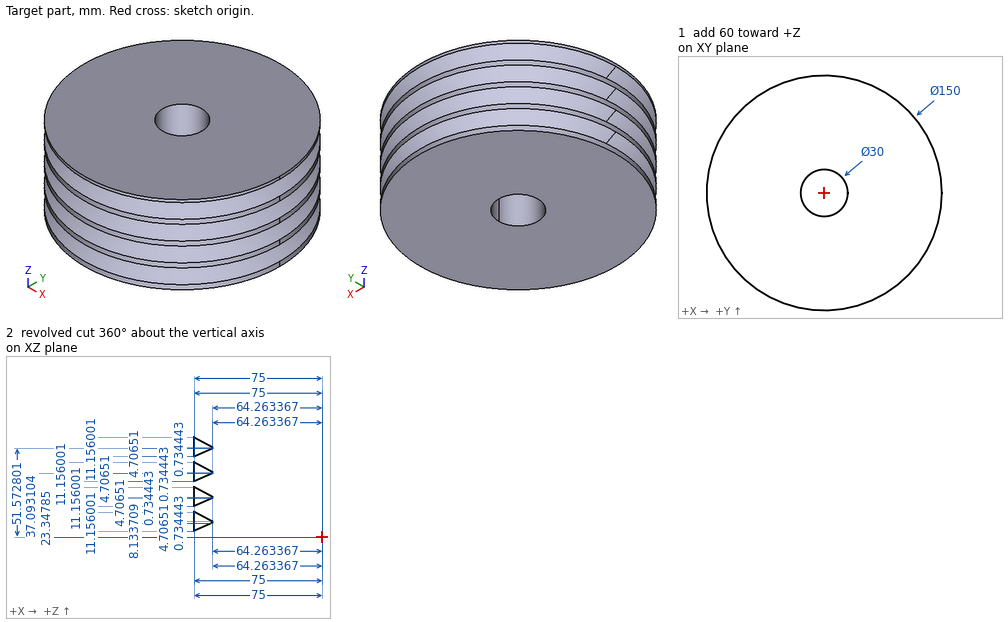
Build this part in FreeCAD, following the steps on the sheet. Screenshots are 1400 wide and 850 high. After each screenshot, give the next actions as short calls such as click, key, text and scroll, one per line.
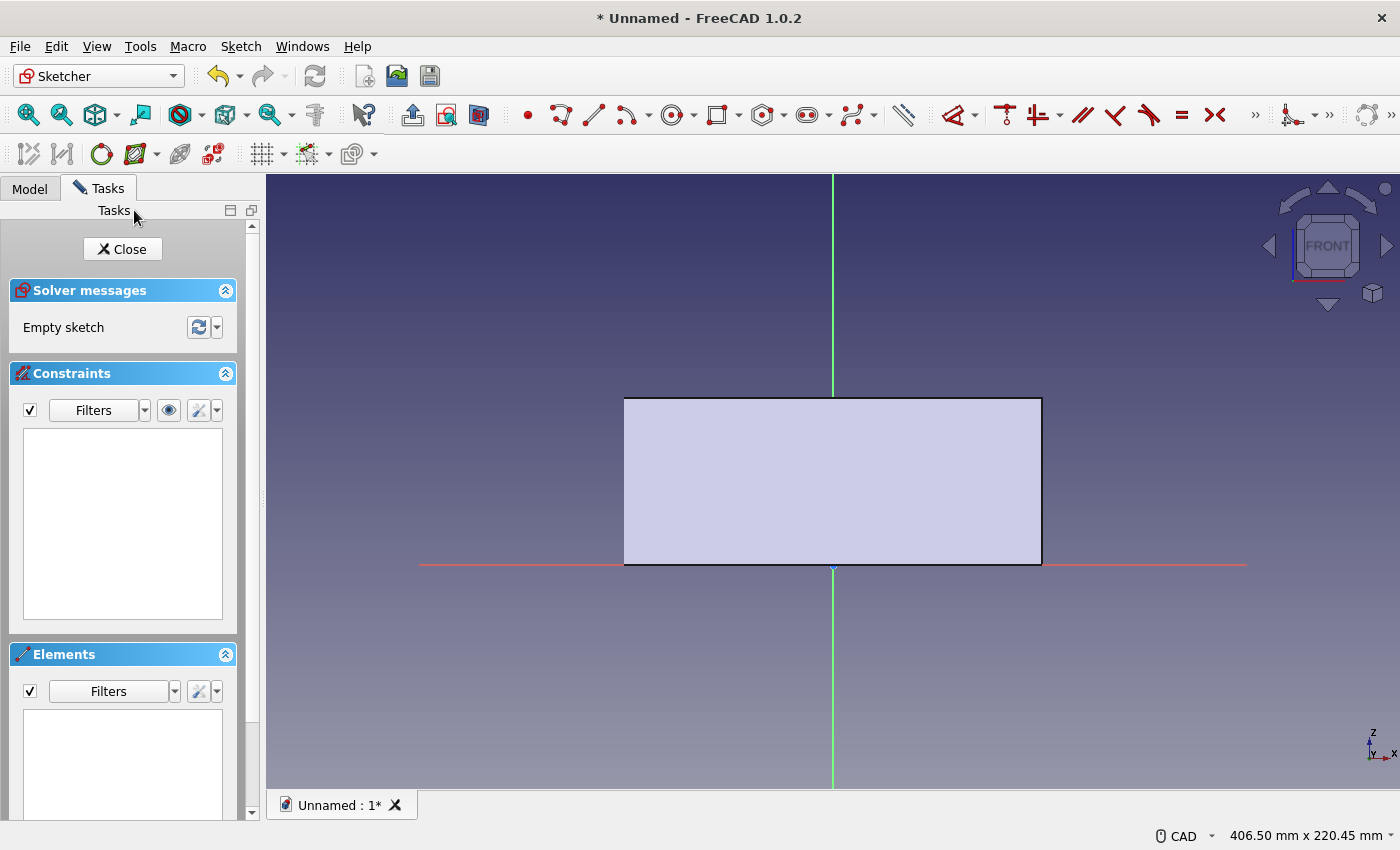
click(479, 116)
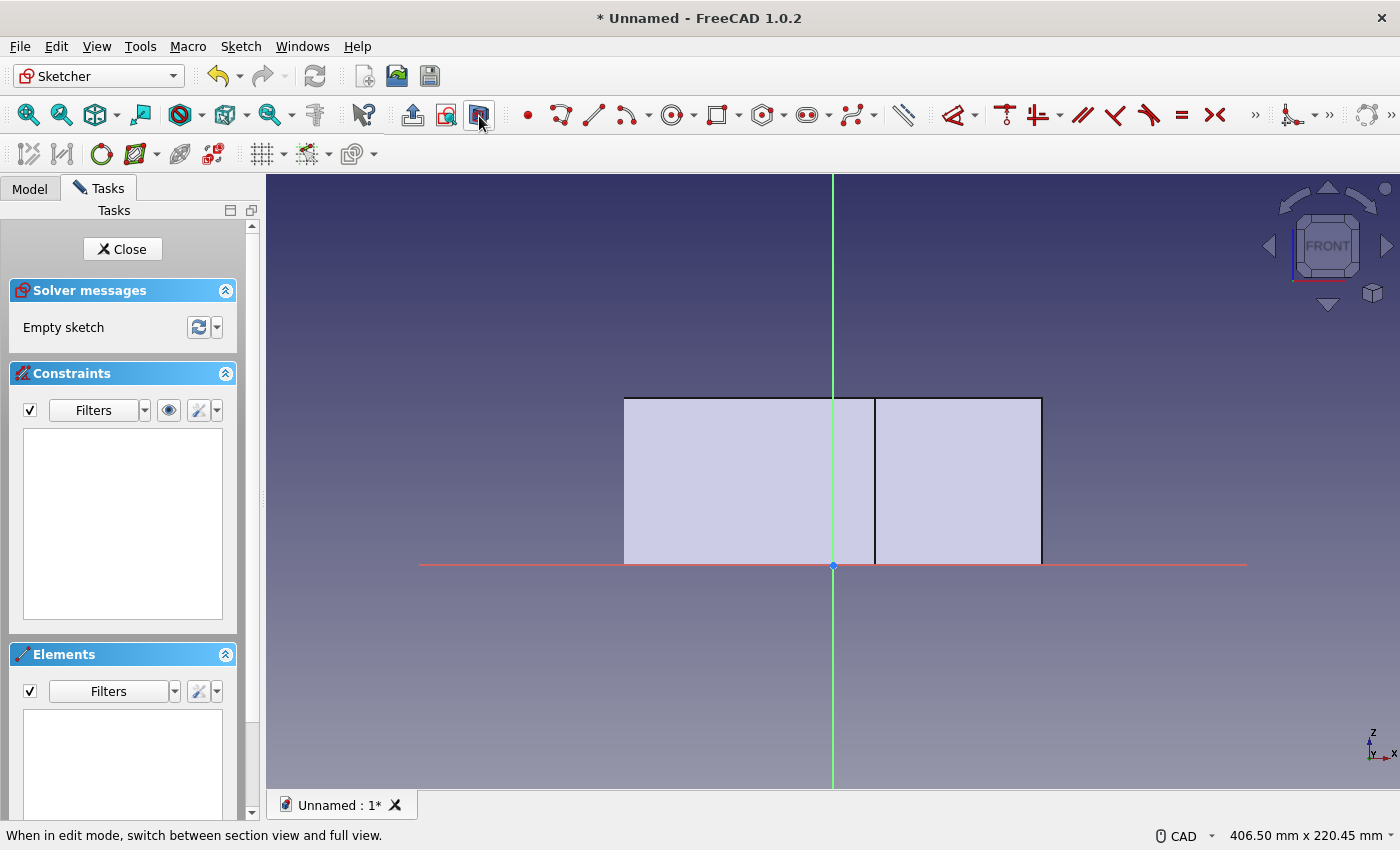
scroll(699, 487, up, 4)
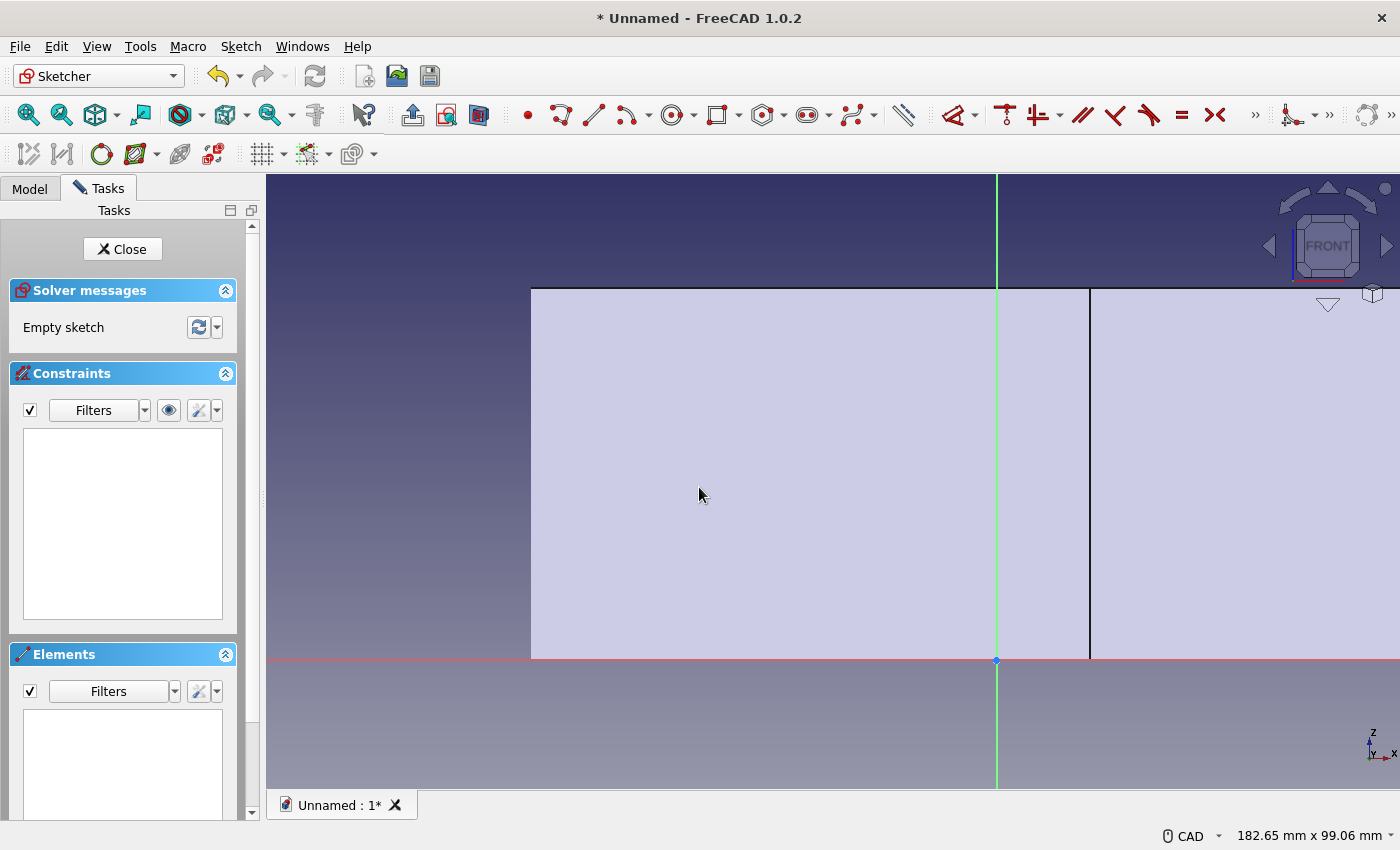
click(561, 116)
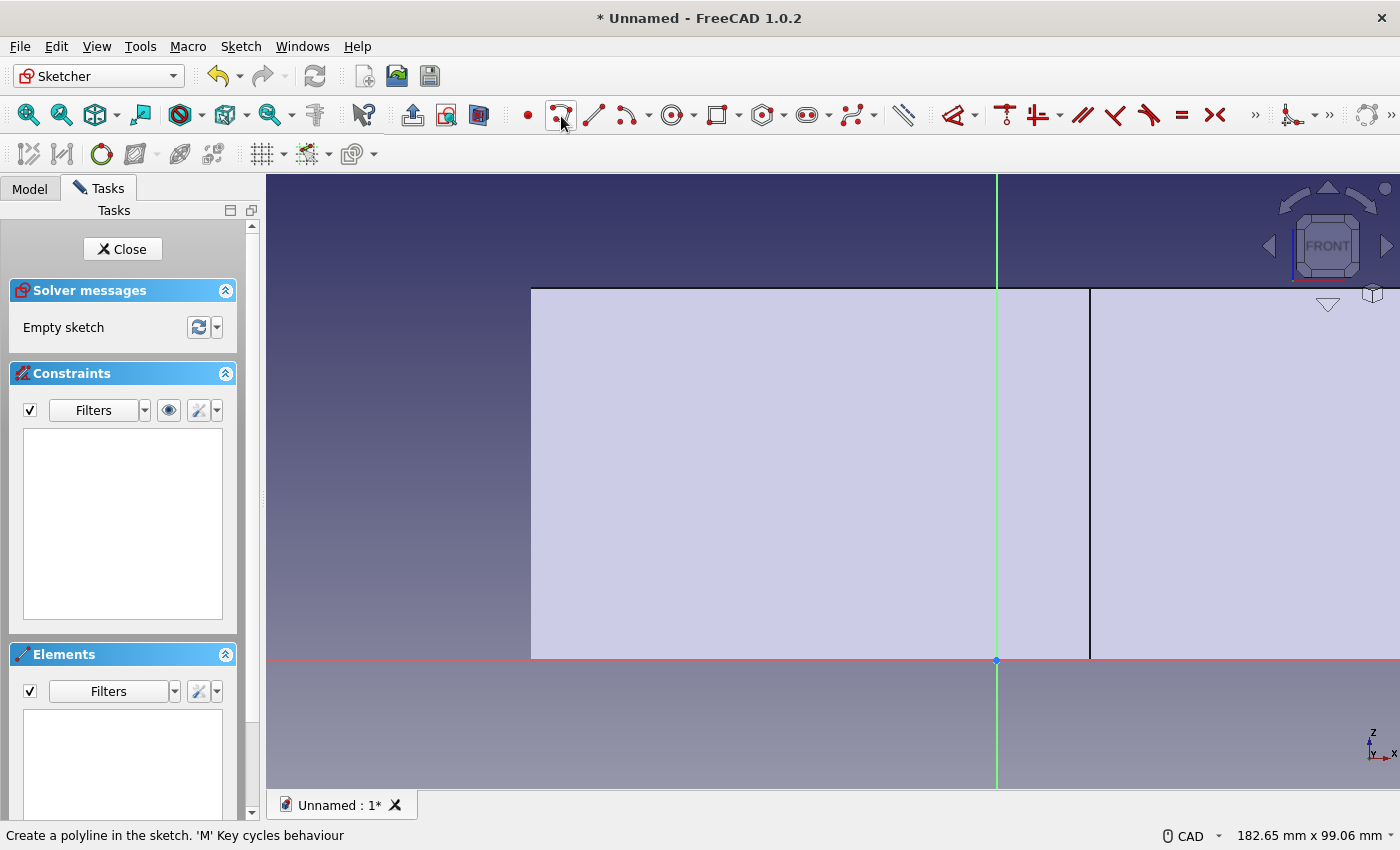
click(598, 340)
click(531, 369)
click(531, 300)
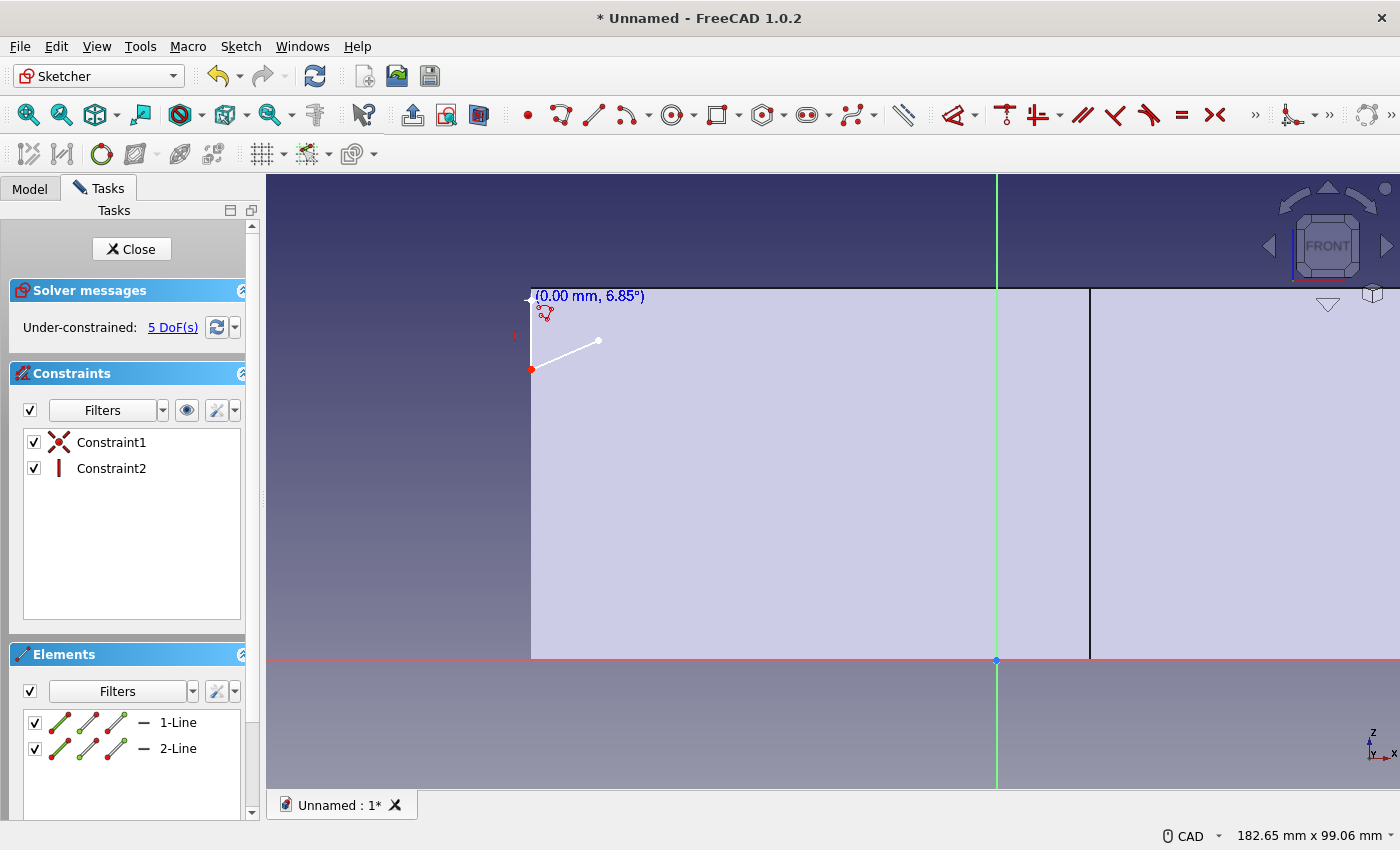
scroll(598, 336, up, 7)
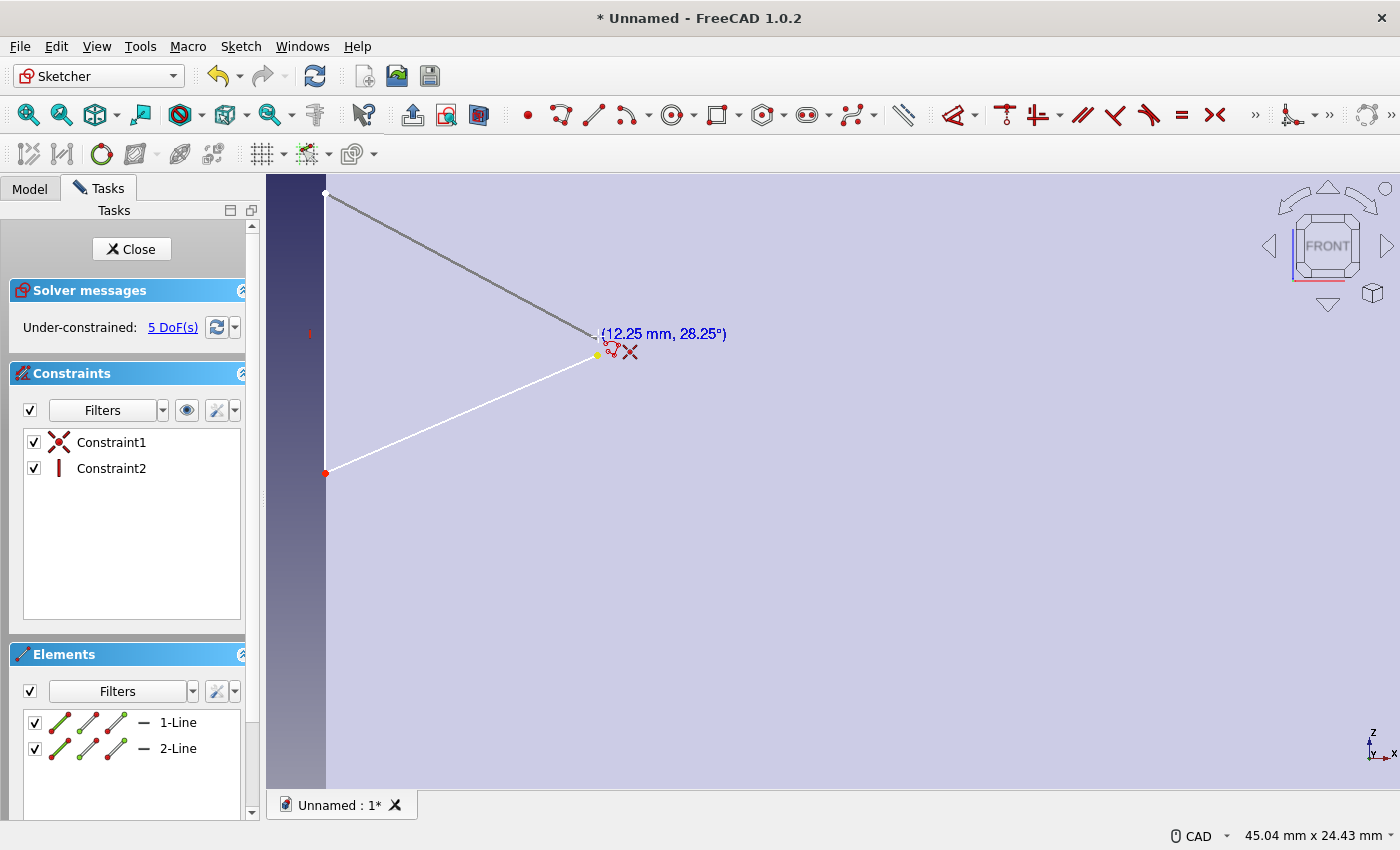
click(596, 334)
click(597, 355)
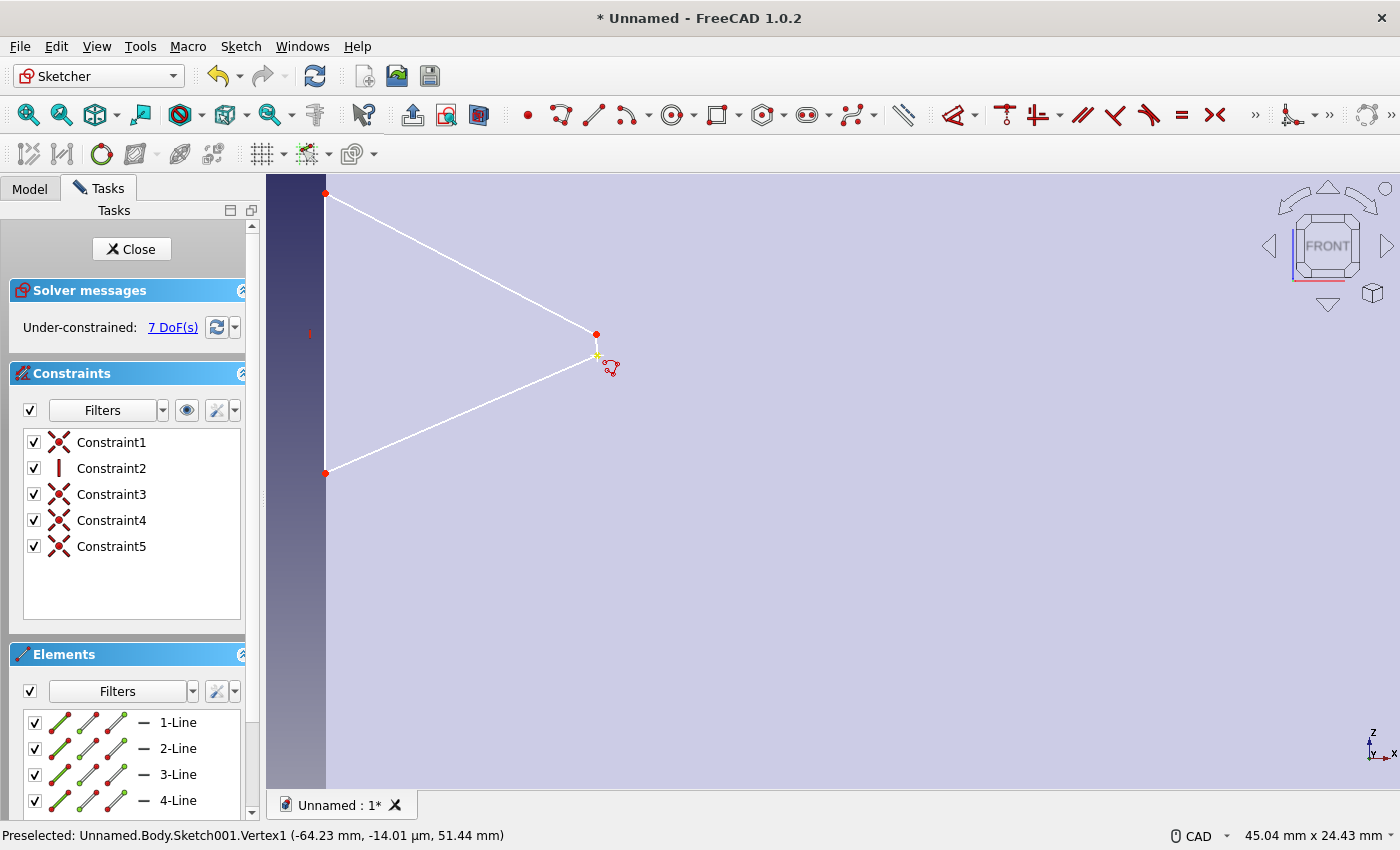
scroll(599, 338, down, 7)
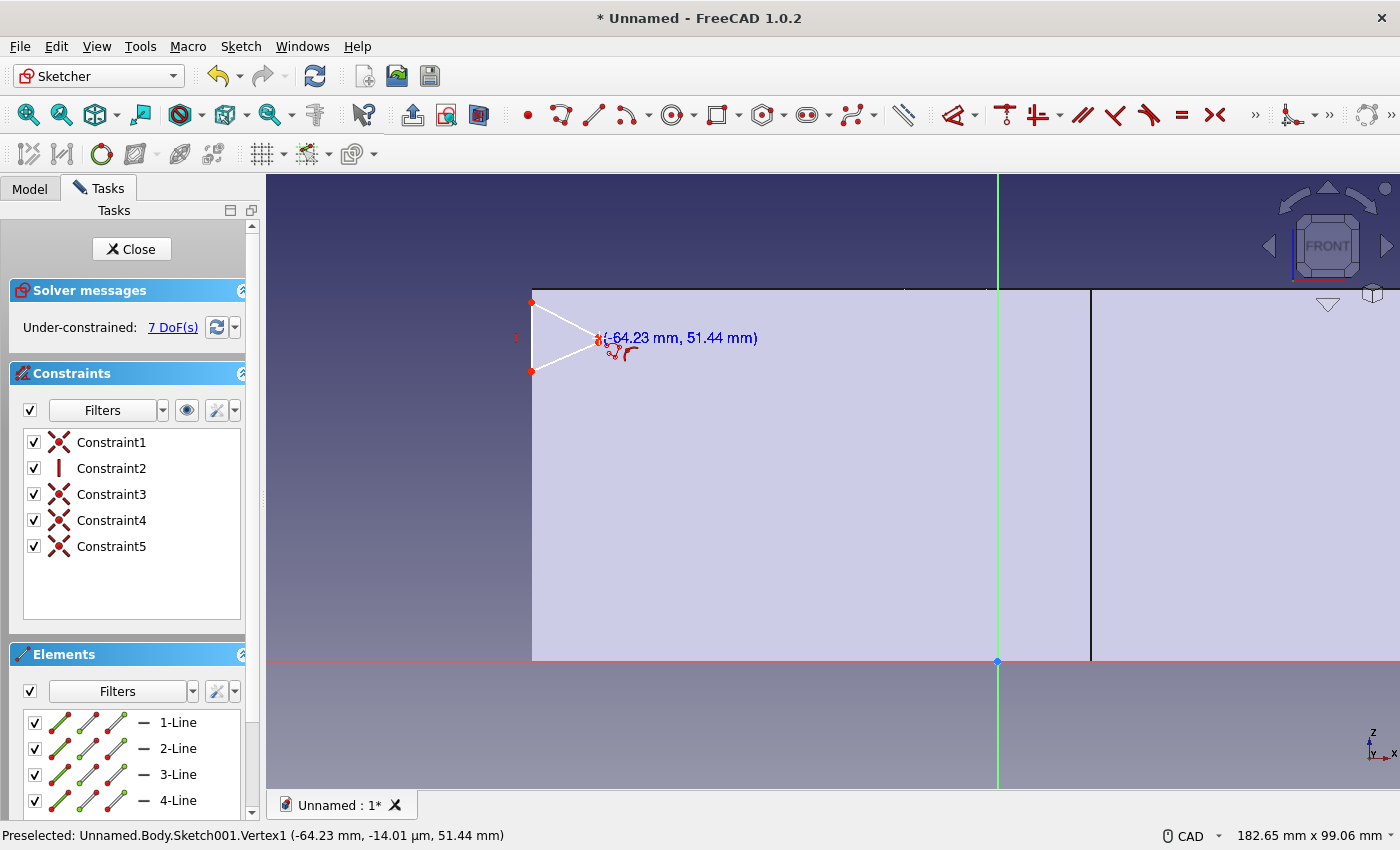
click(599, 432)
click(532, 461)
click(532, 392)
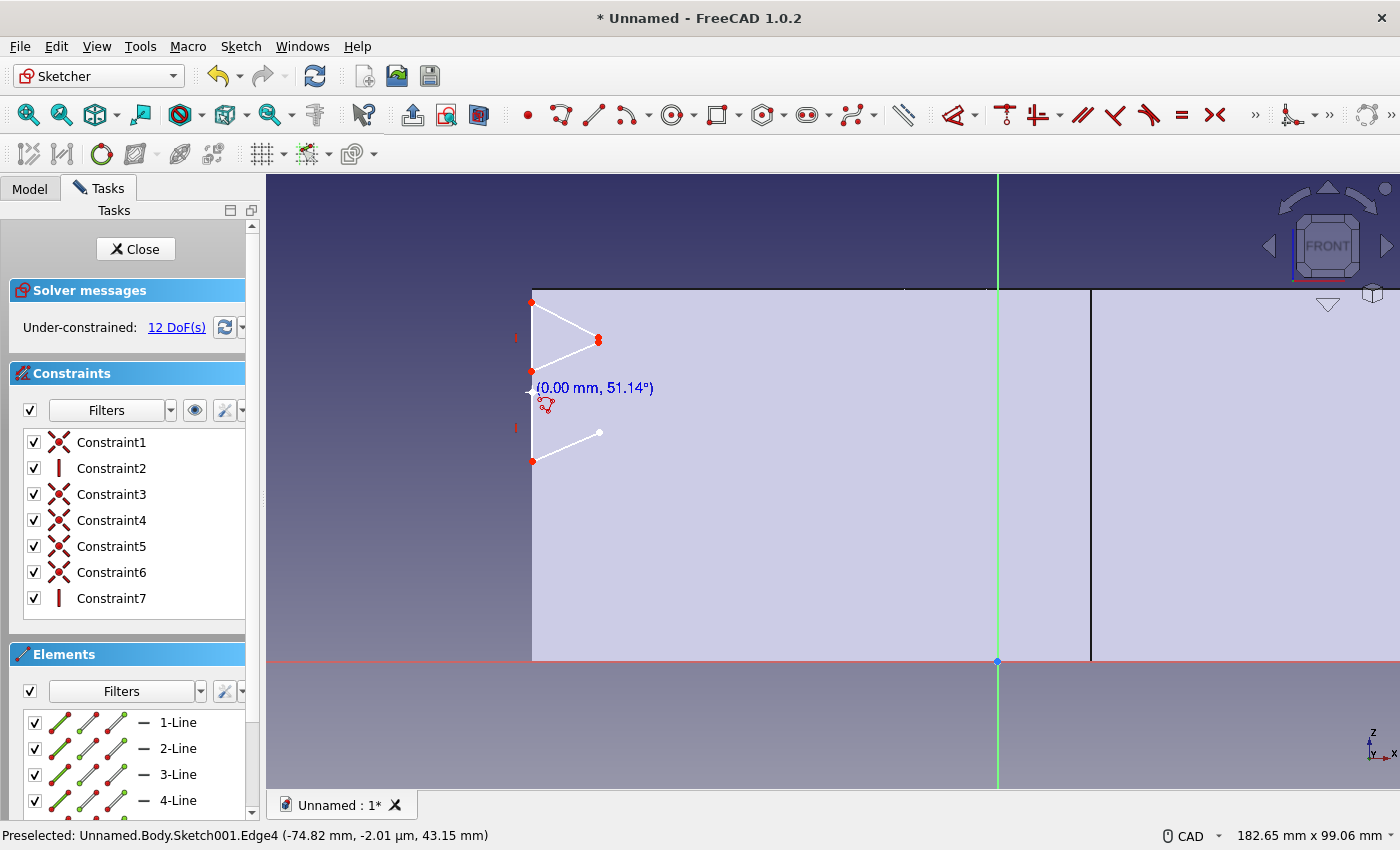
scroll(599, 427, up, 7)